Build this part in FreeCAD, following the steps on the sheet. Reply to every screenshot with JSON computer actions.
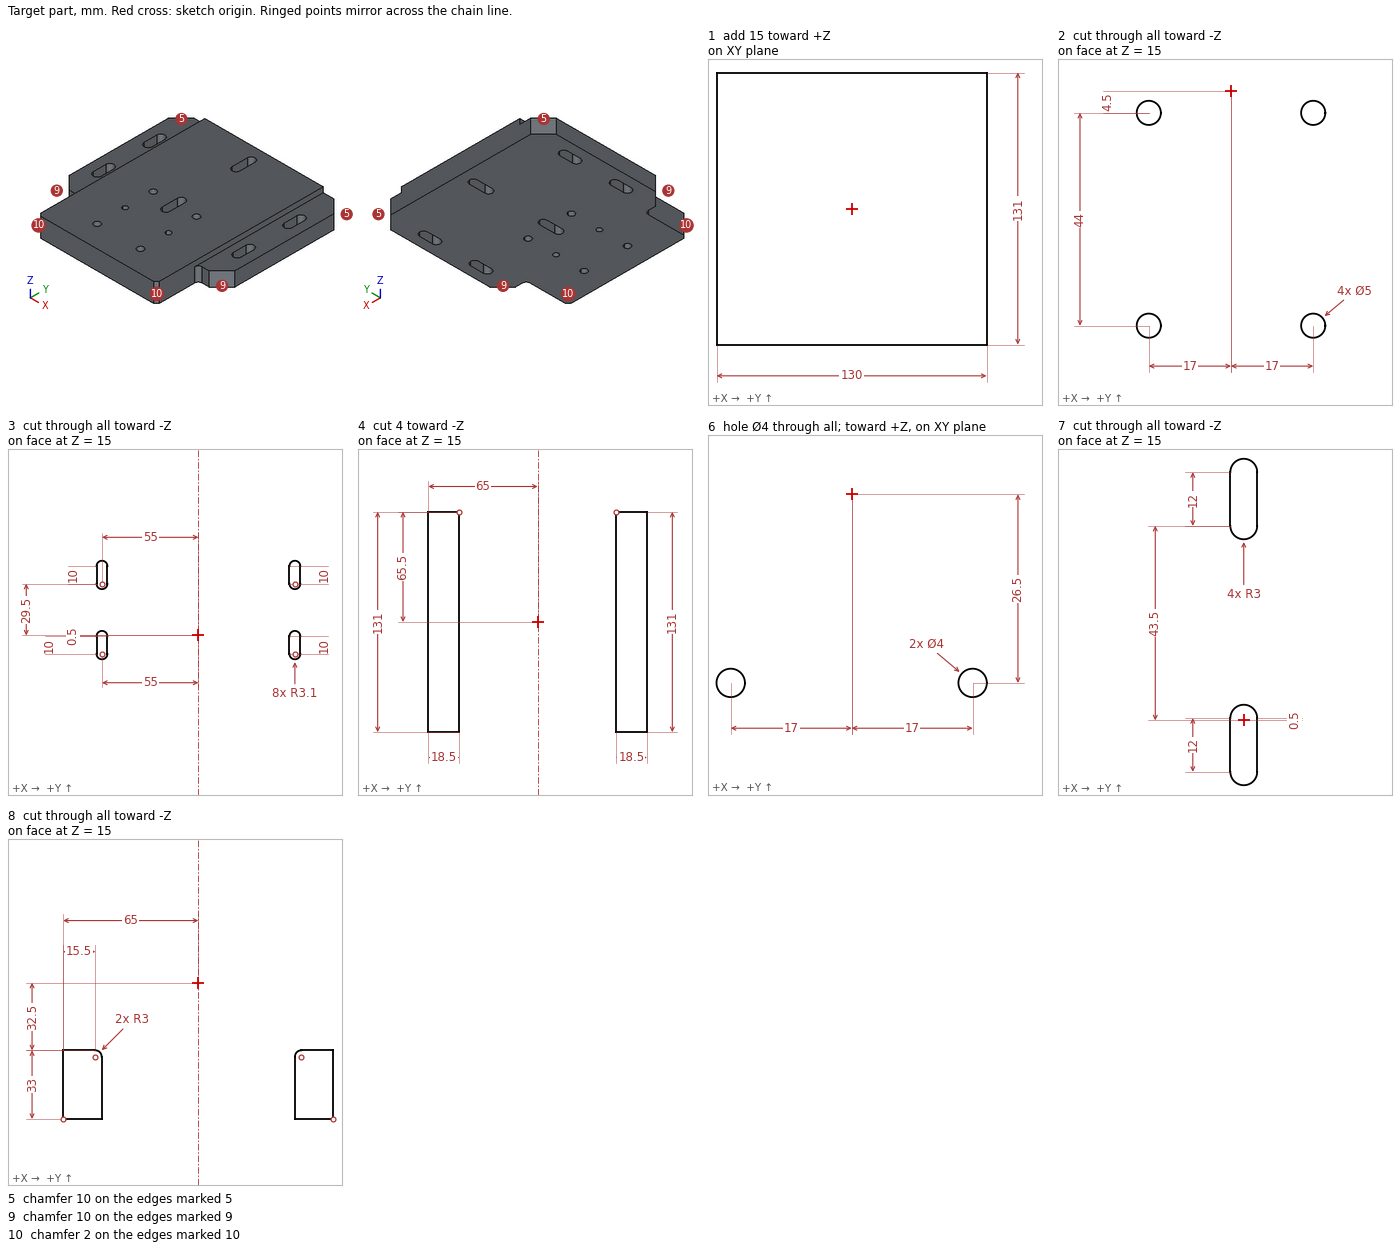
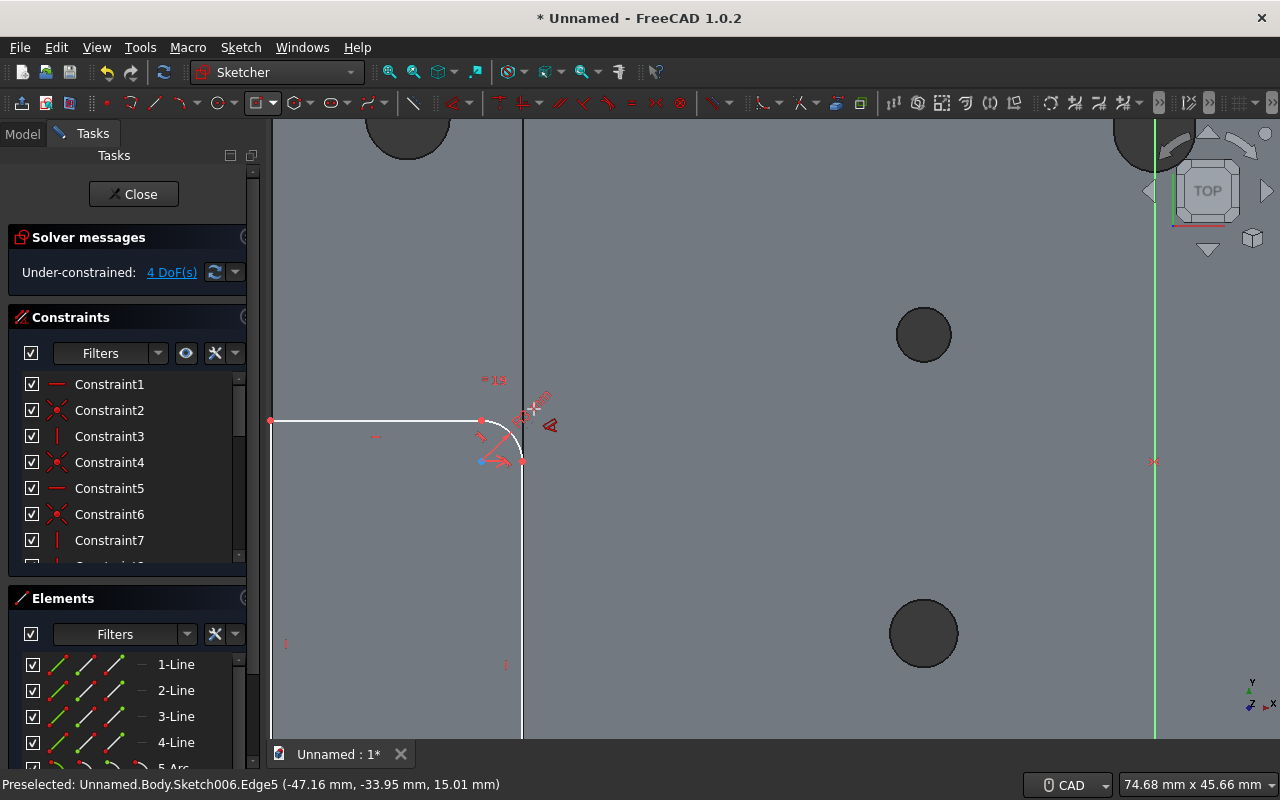
{"action": "scroll", "coordinate": [510, 433], "scroll_direction": "down", "scroll_amount": 6}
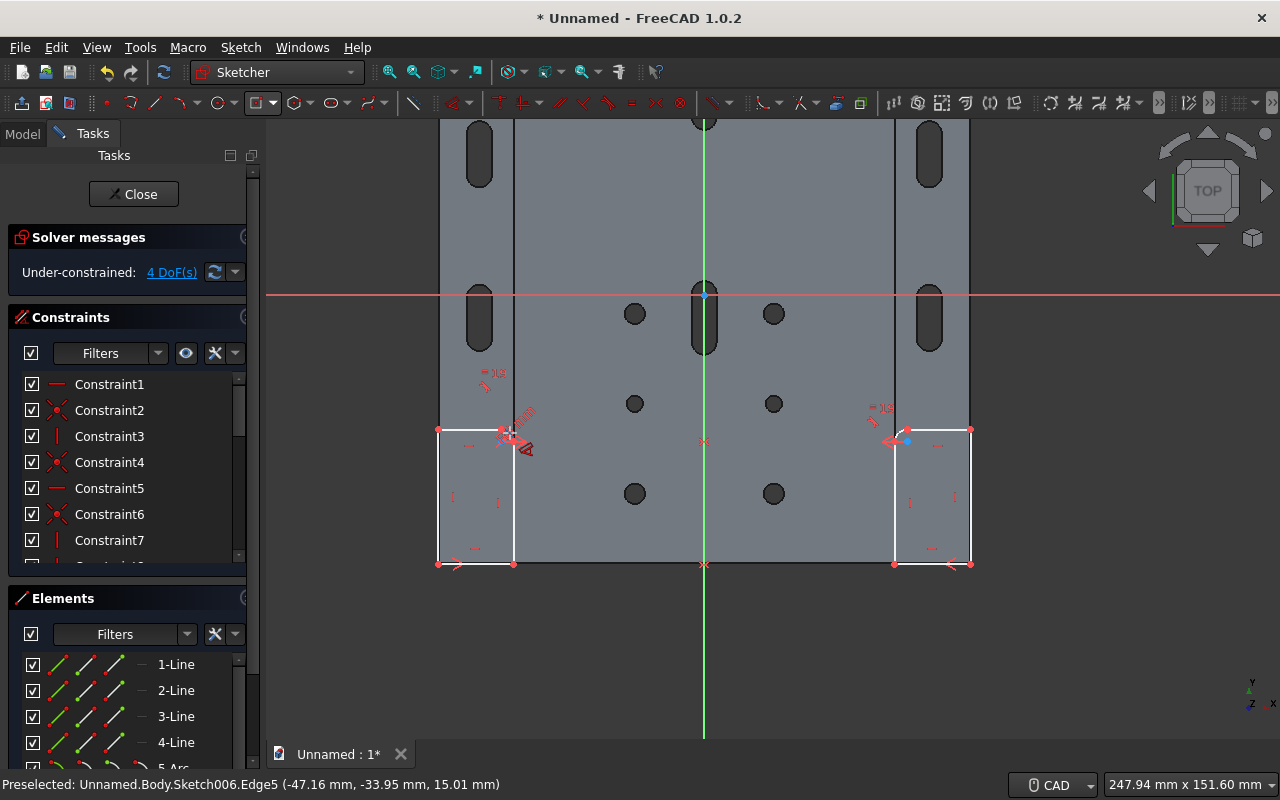
{"action": "left_click", "coordinate": [438, 470]}
{"action": "left_click", "coordinate": [404, 497]}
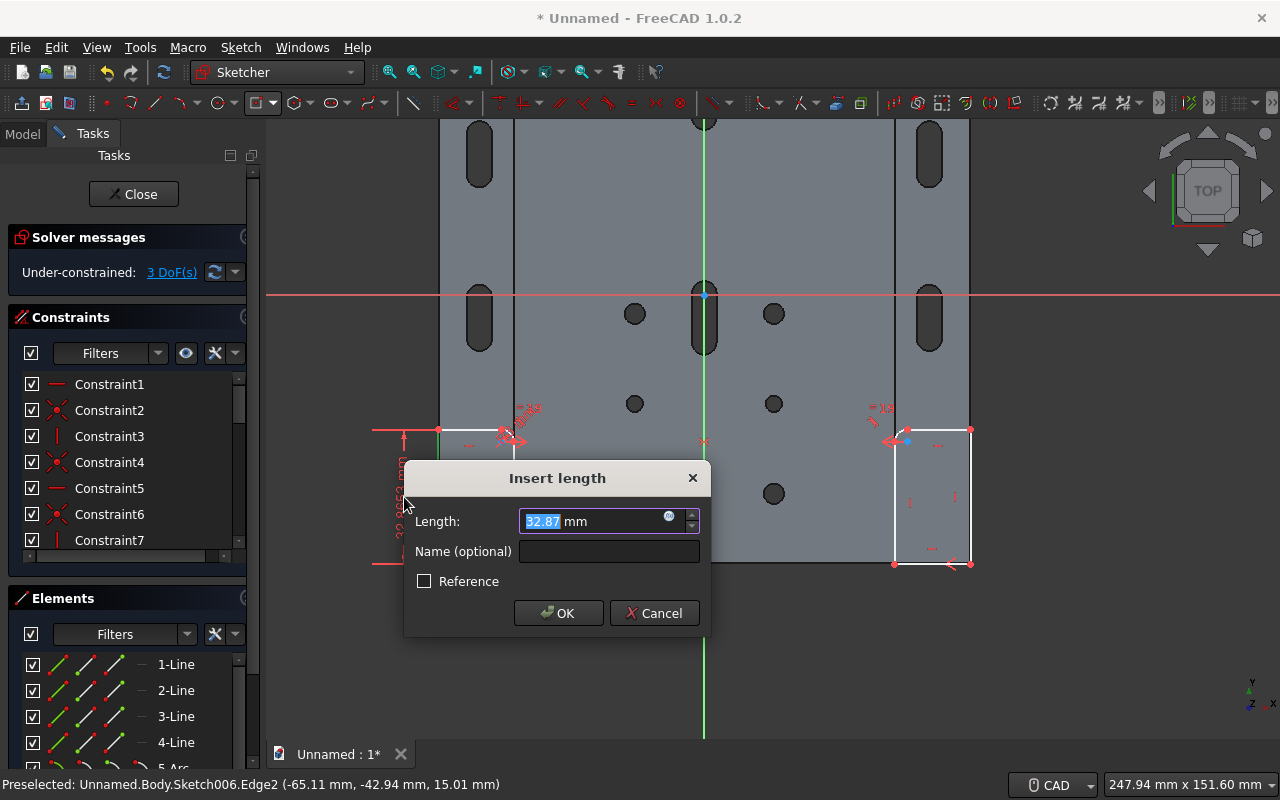
{"action": "type", "text": "33"}
{"action": "key", "text": "Return"}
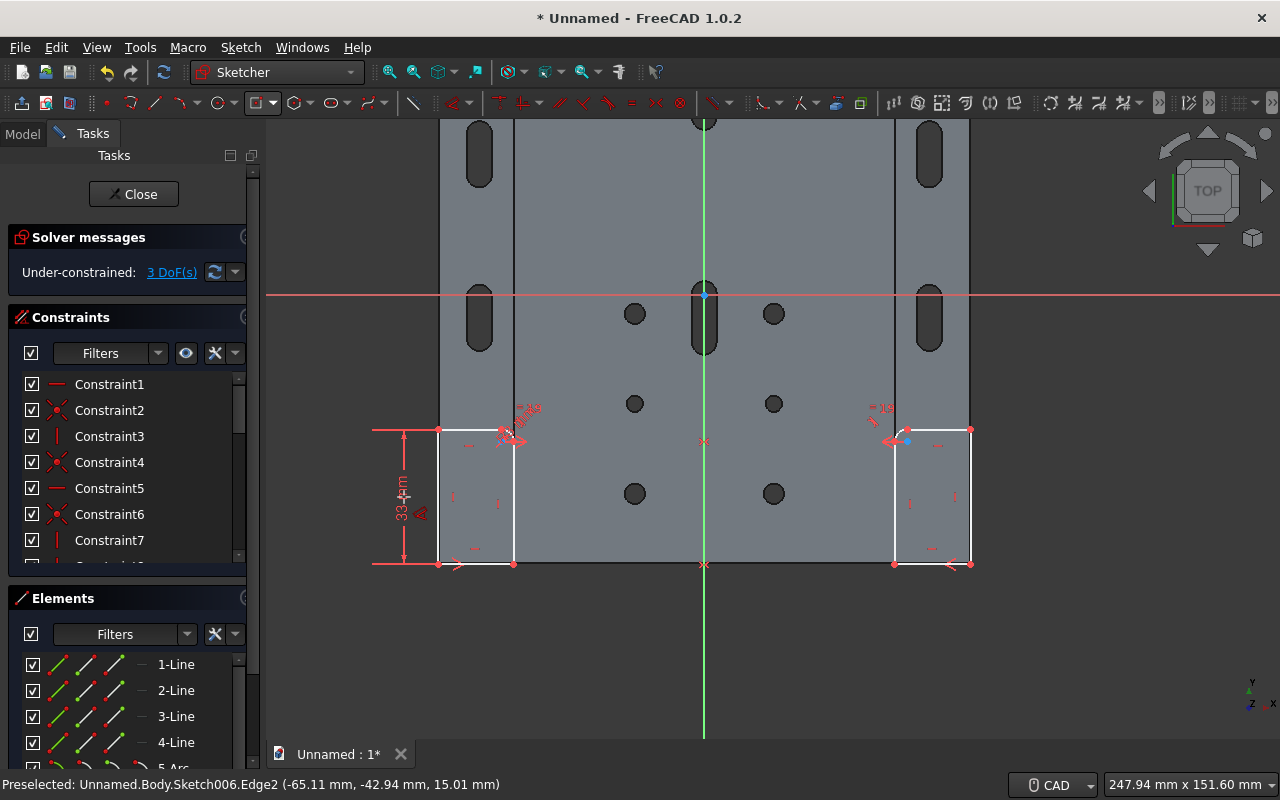
{"action": "left_click", "coordinate": [438, 430]}
{"action": "left_click", "coordinate": [571, 261]}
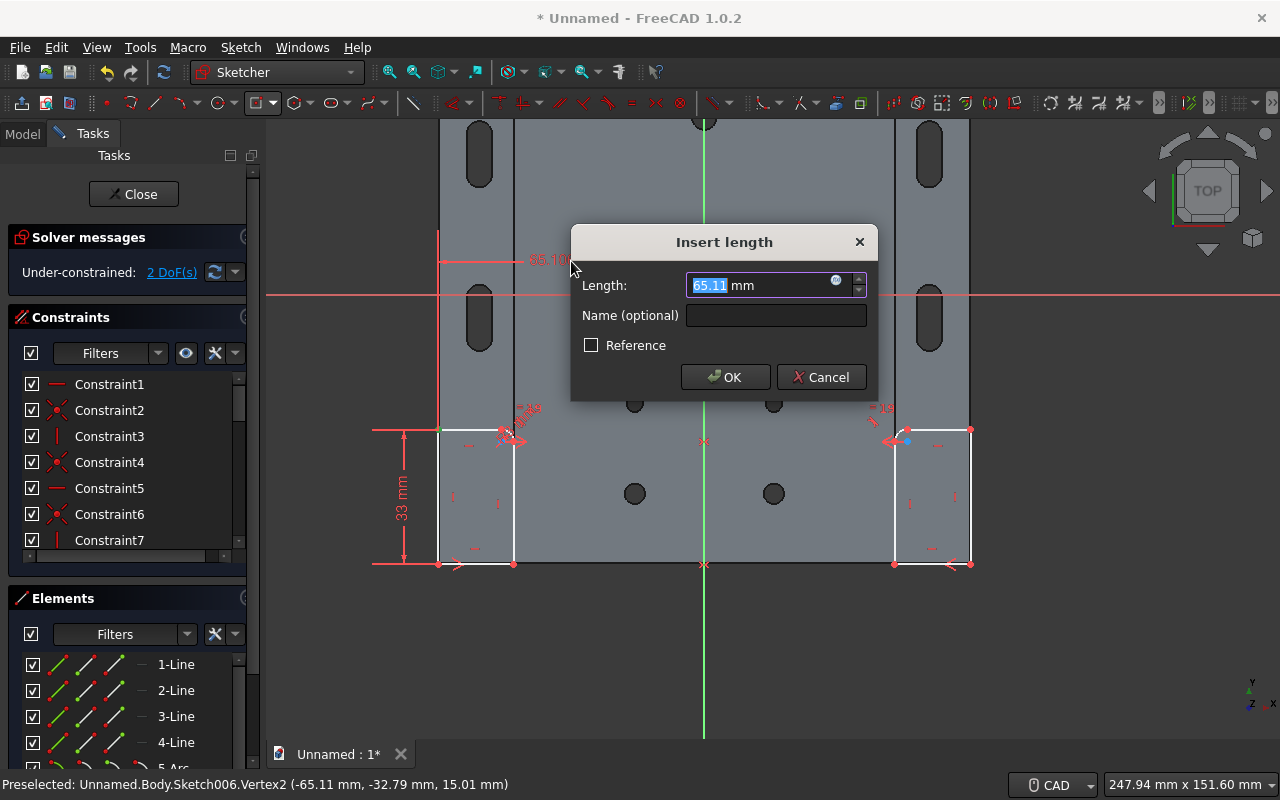
{"action": "type", "text": "65"}
{"action": "key", "text": "Return"}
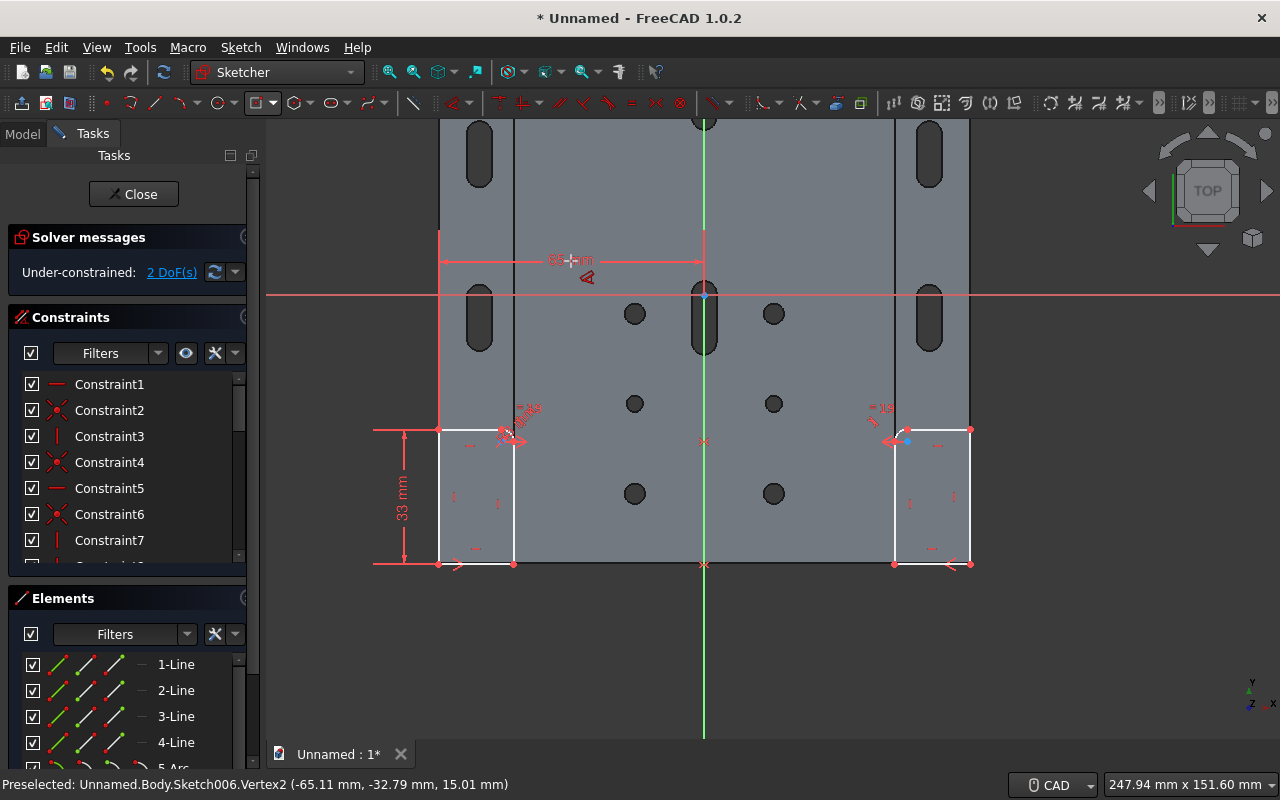
{"action": "left_click", "coordinate": [483, 430]}
{"action": "left_click", "coordinate": [470, 464]}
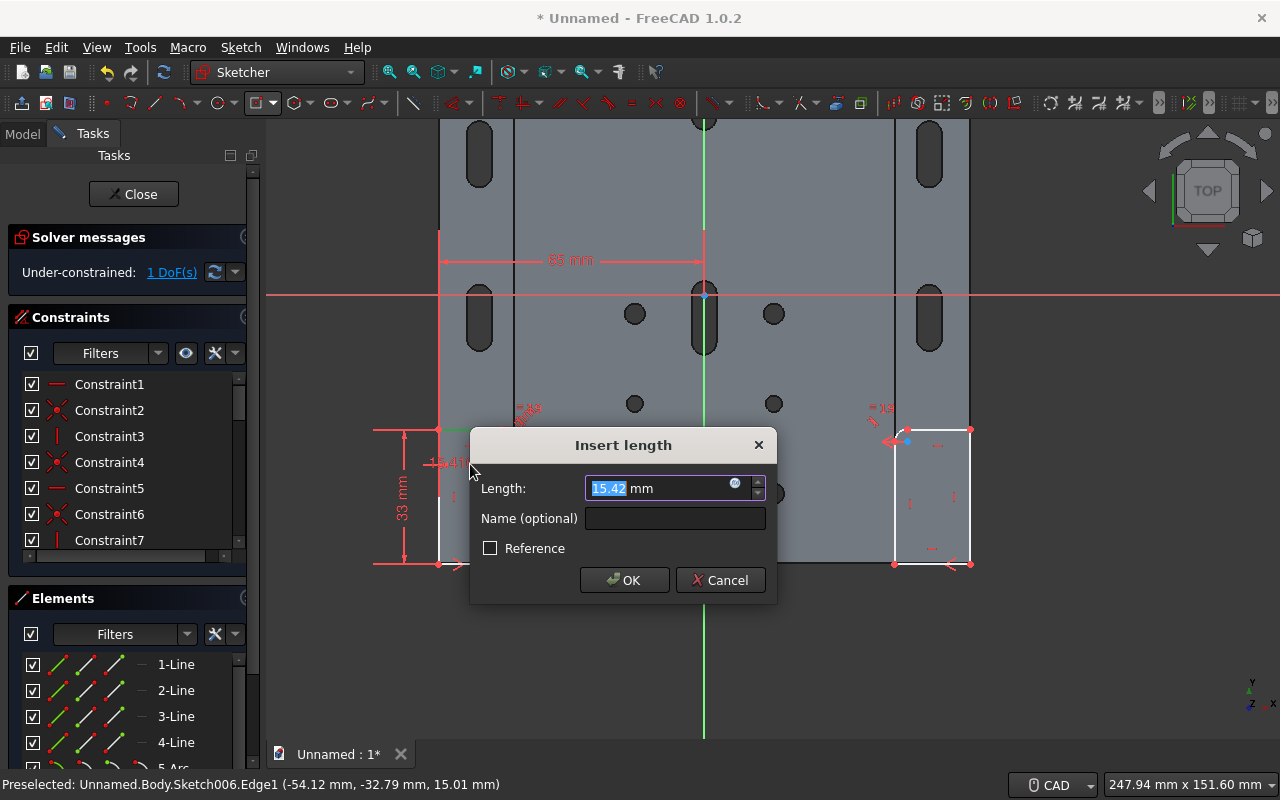
{"action": "type", "text": "15.5"}
{"action": "key", "text": "Return"}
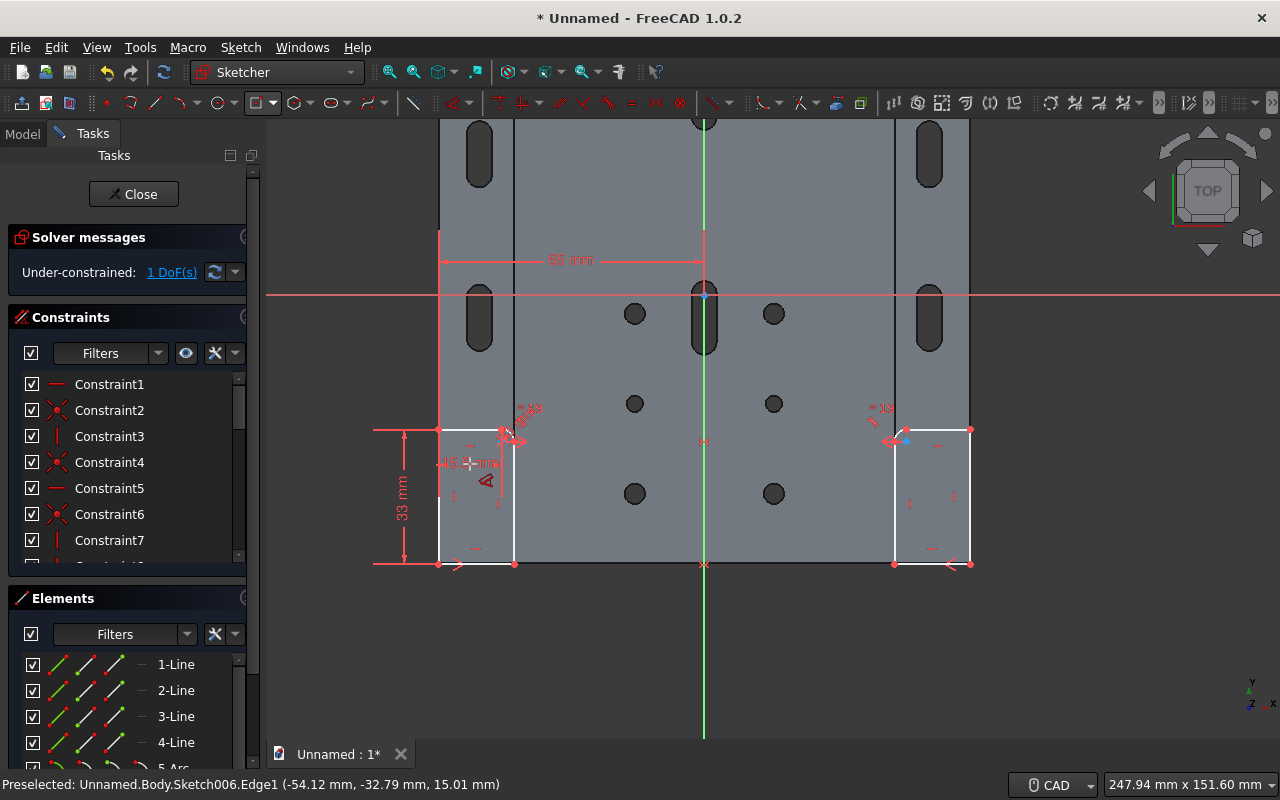
{"action": "left_click", "coordinate": [502, 430]}
{"action": "left_click", "coordinate": [468, 362]}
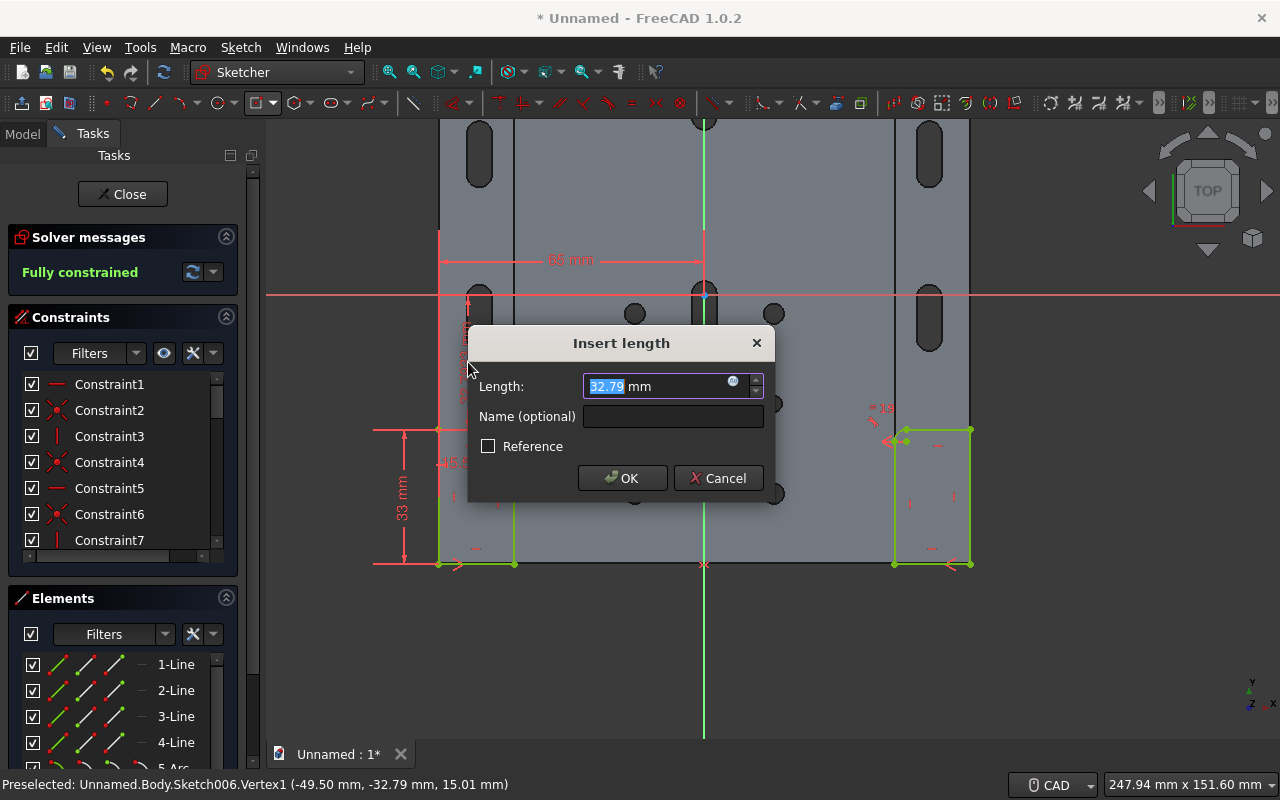
{"action": "type", "text": "32.5"}
{"action": "key", "text": "Return"}
{"action": "key", "text": "Escape"}